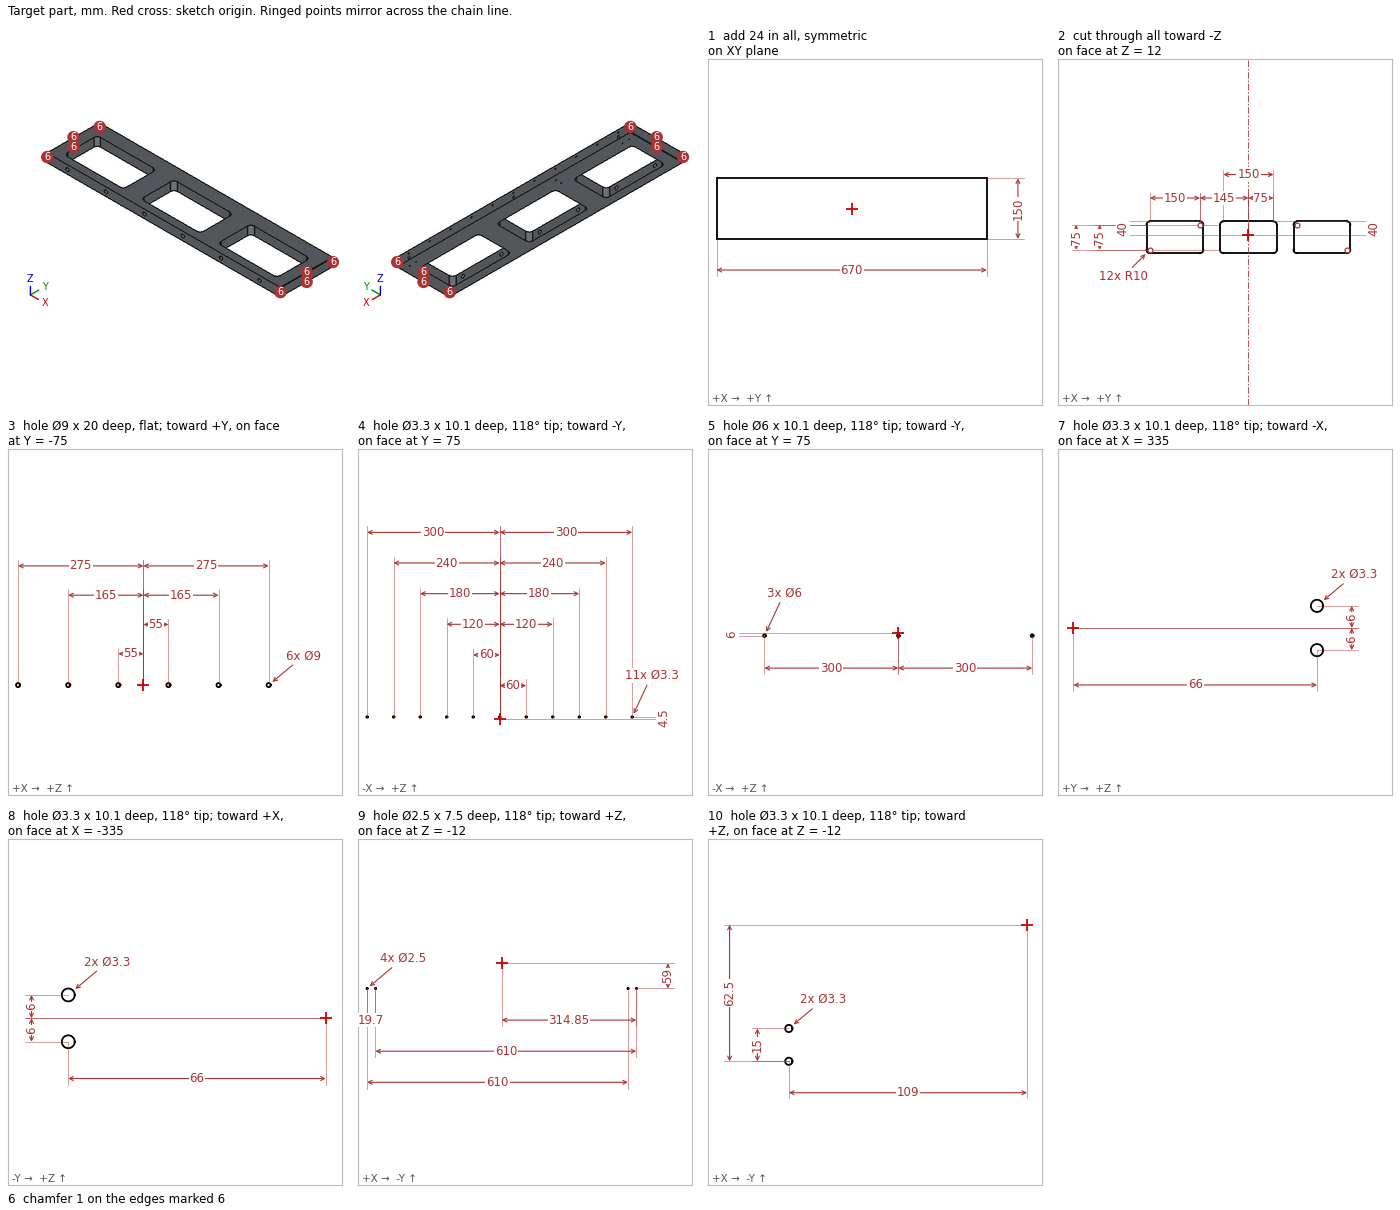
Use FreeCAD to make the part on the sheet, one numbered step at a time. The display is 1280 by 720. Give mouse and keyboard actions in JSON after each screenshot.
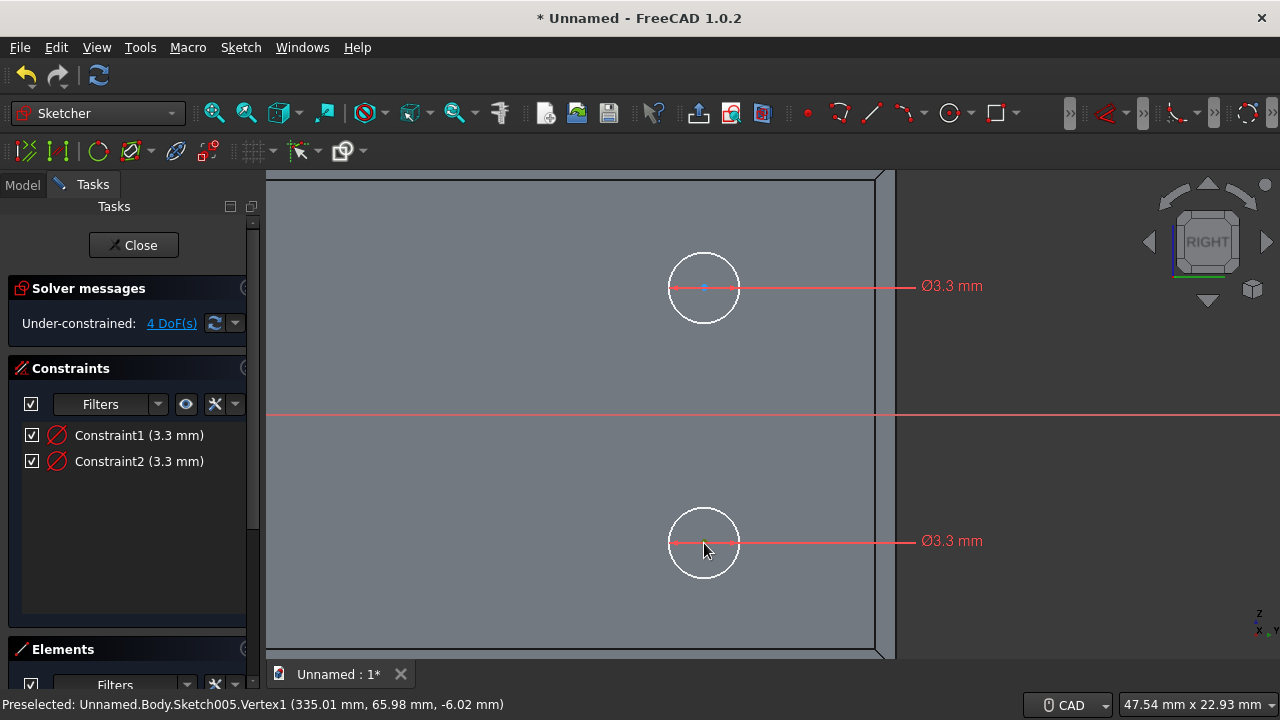
{"action": "left_click", "coordinate": [704, 288]}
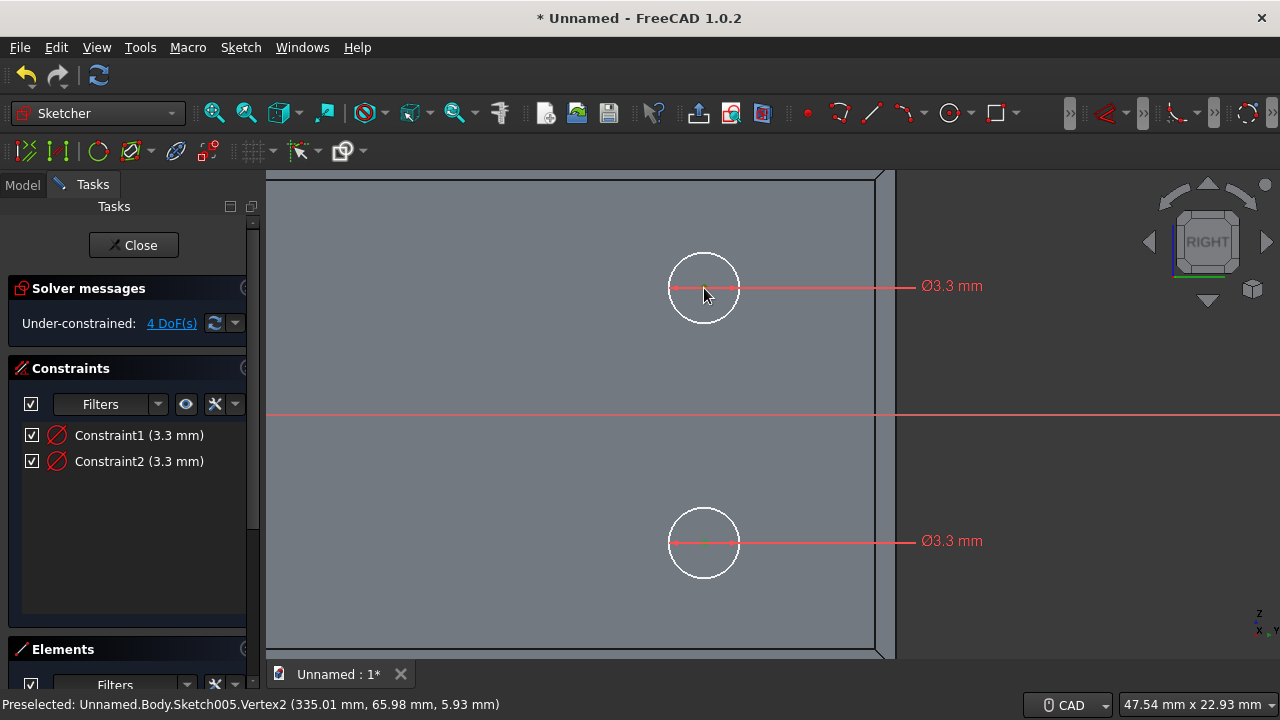
{"action": "key", "text": "v"}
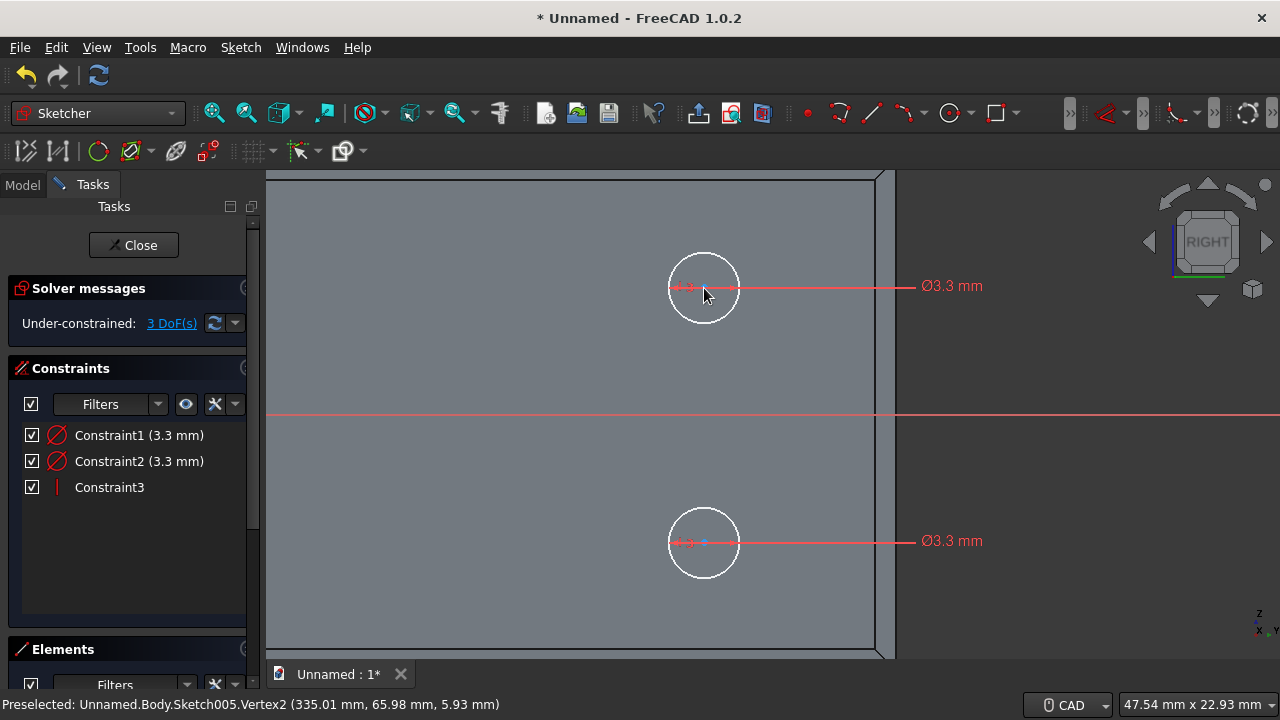
{"action": "left_click", "coordinate": [1106, 114]}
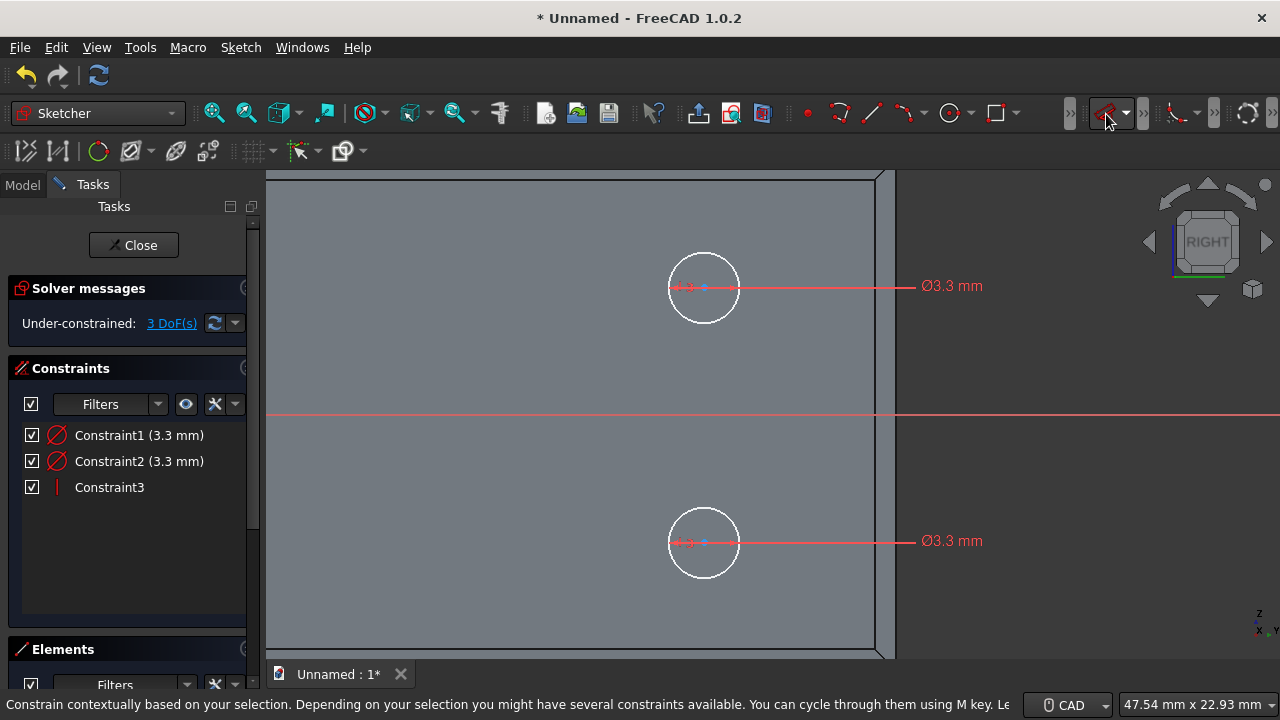
{"action": "left_click", "coordinate": [704, 543]}
{"action": "left_click", "coordinate": [738, 479]}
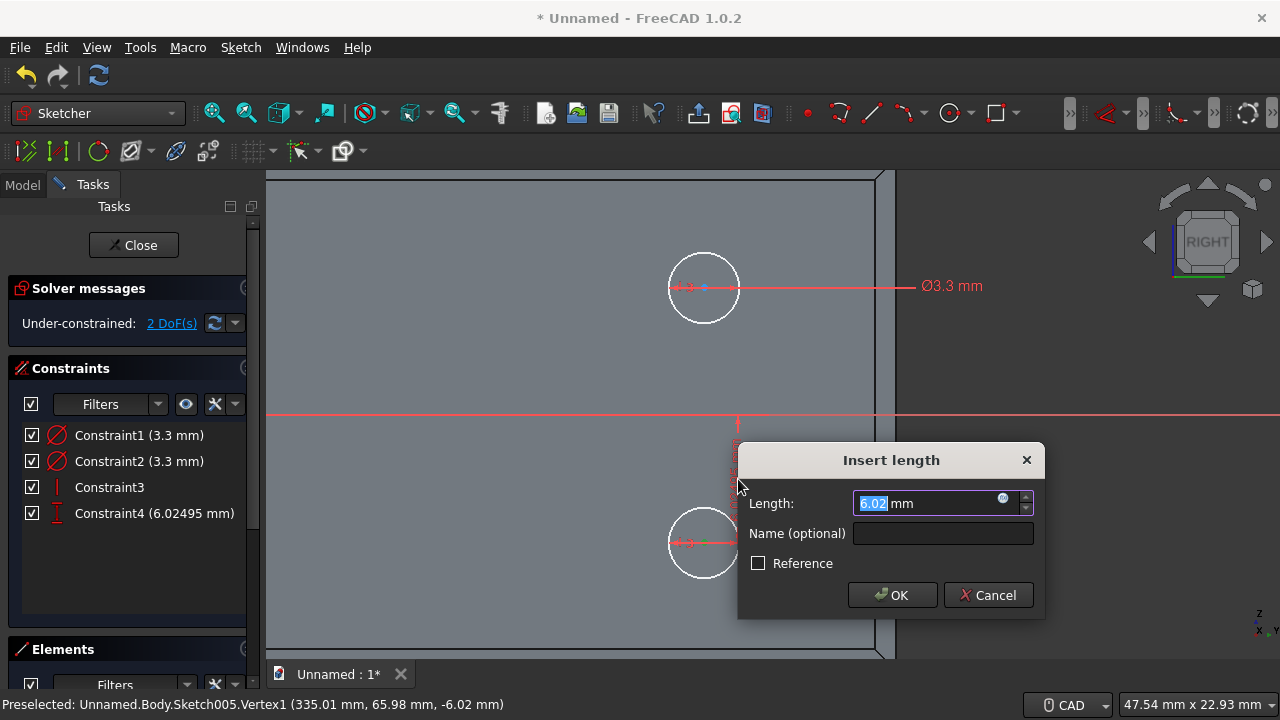
{"action": "type", "text": "6"}
{"action": "key", "text": "Return"}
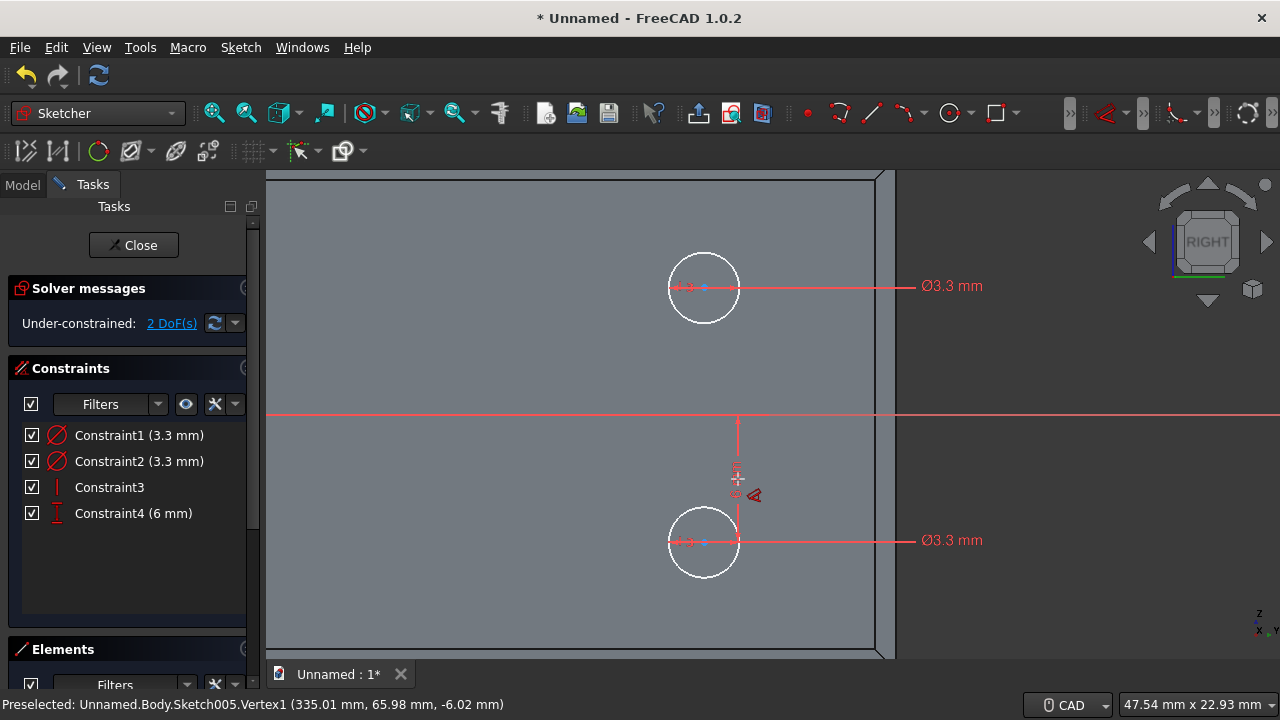
{"action": "left_click", "coordinate": [704, 288]}
{"action": "left_click", "coordinate": [738, 351]}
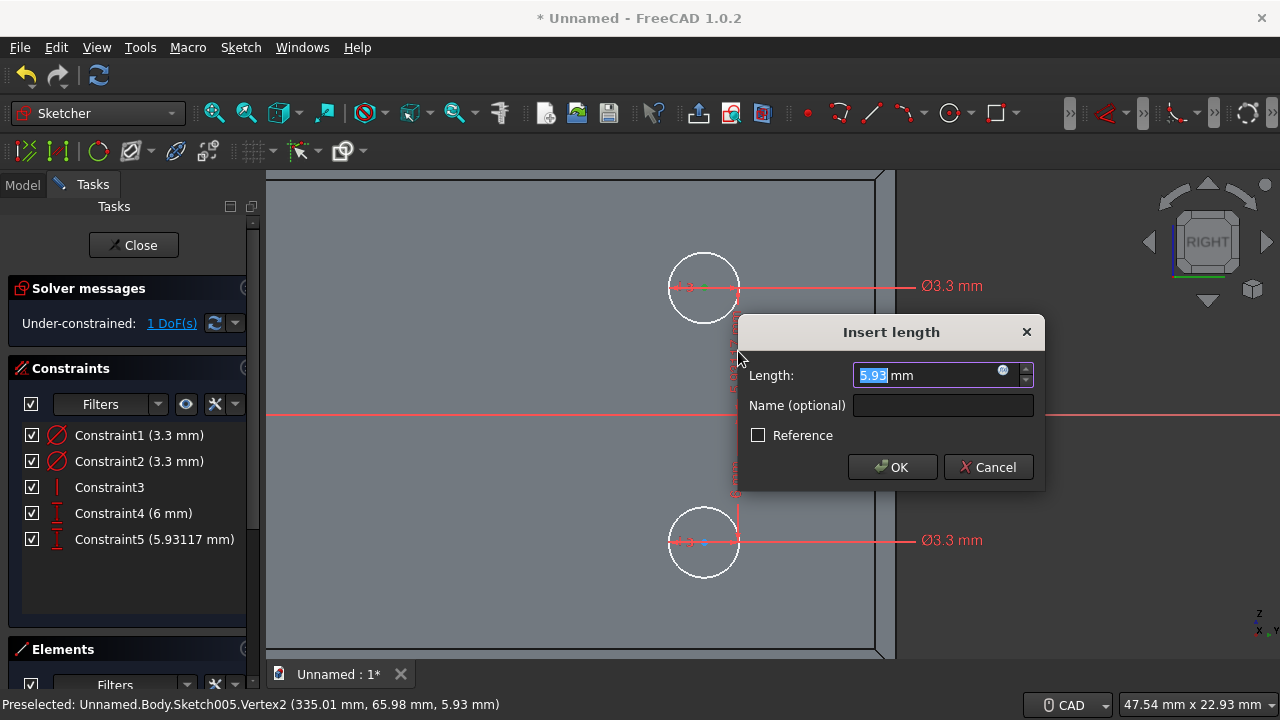
{"action": "type", "text": "6"}
{"action": "key", "text": "Return"}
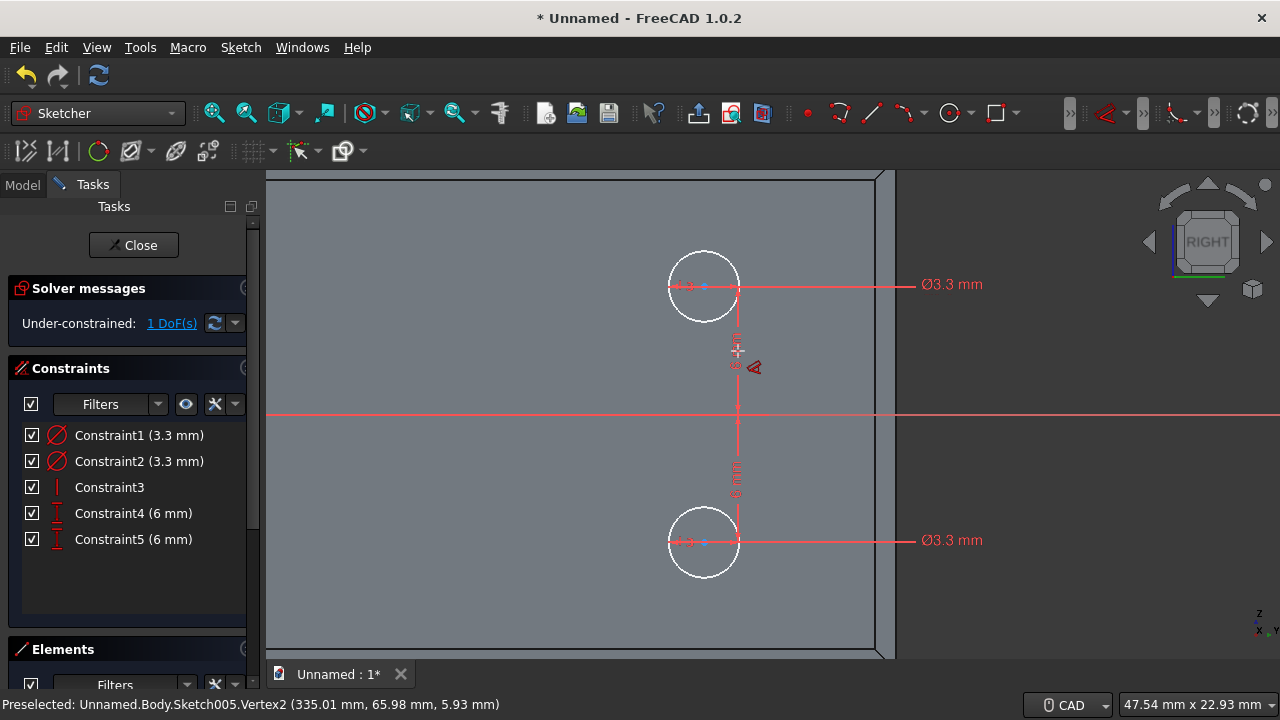
{"action": "left_click", "coordinate": [704, 542]}
{"action": "left_click", "coordinate": [499, 576]}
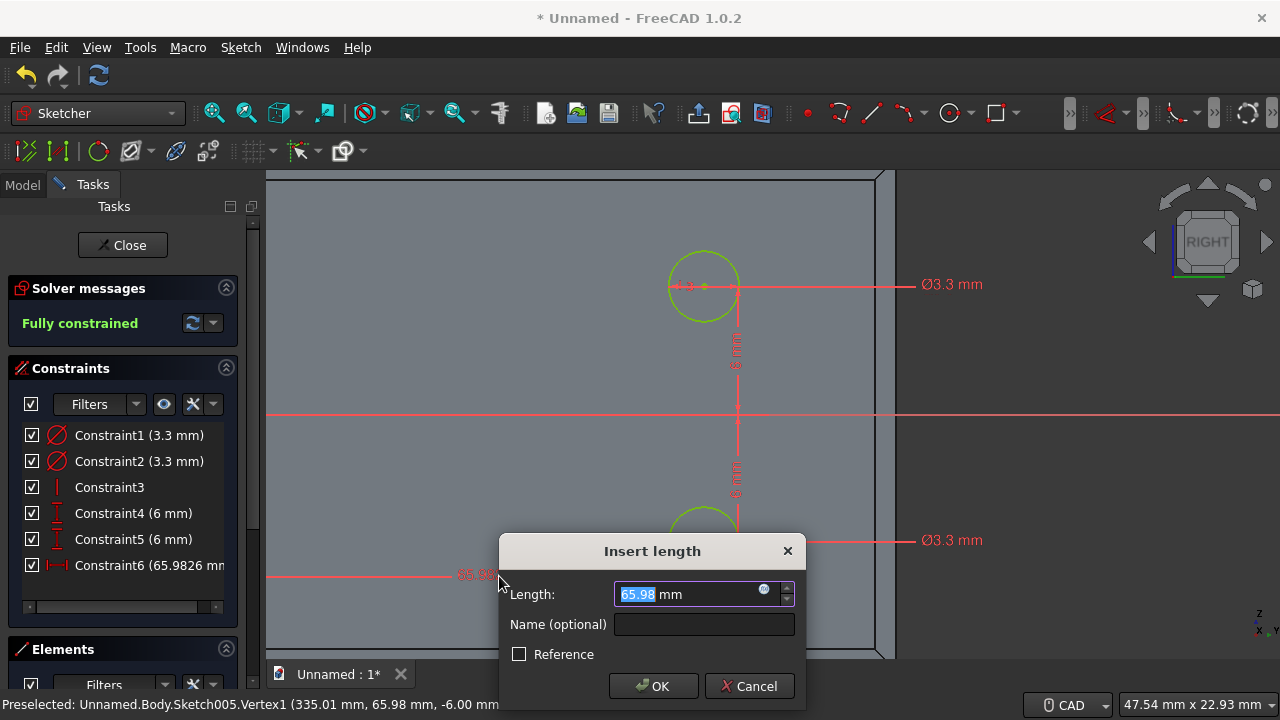
{"action": "type", "text": "66"}
{"action": "key", "text": "Return"}
{"action": "key", "text": "Escape"}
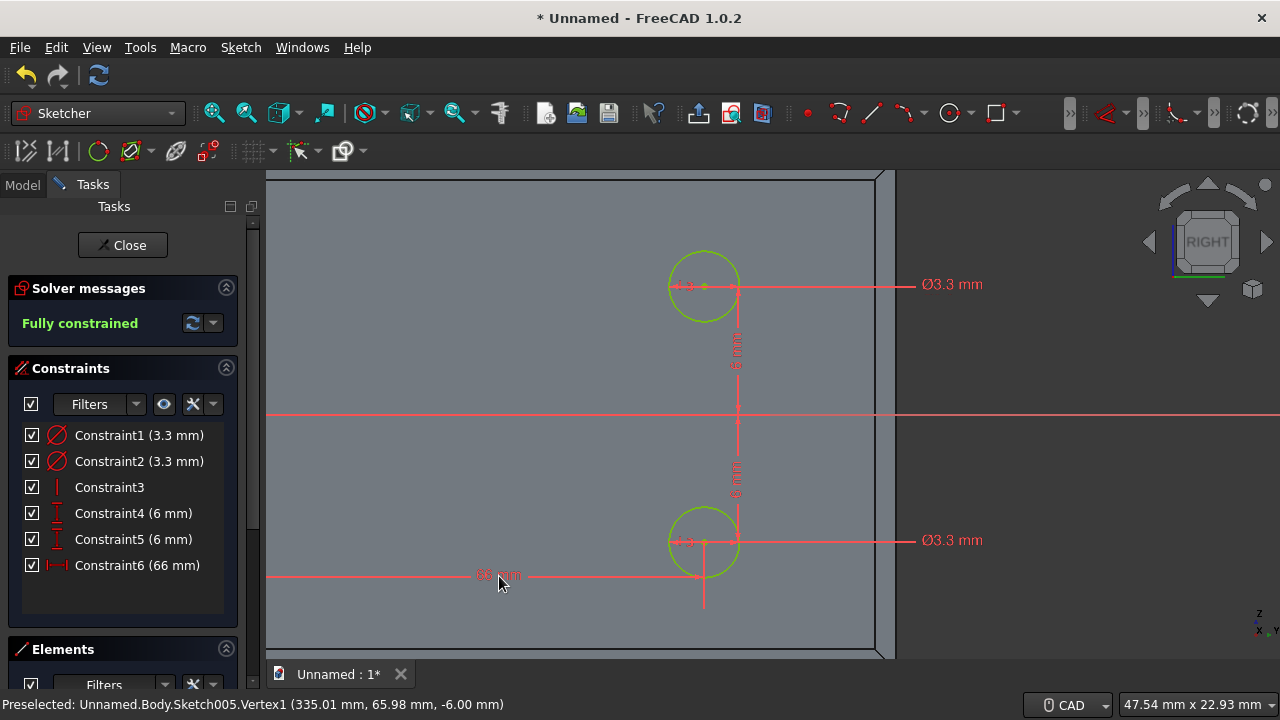
{"action": "left_click", "coordinate": [123, 245]}